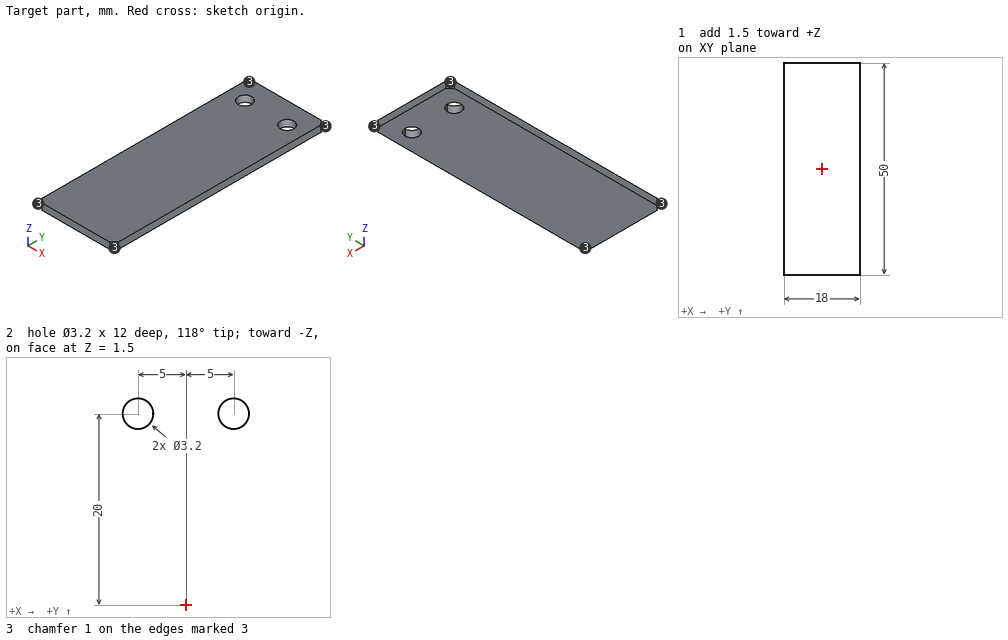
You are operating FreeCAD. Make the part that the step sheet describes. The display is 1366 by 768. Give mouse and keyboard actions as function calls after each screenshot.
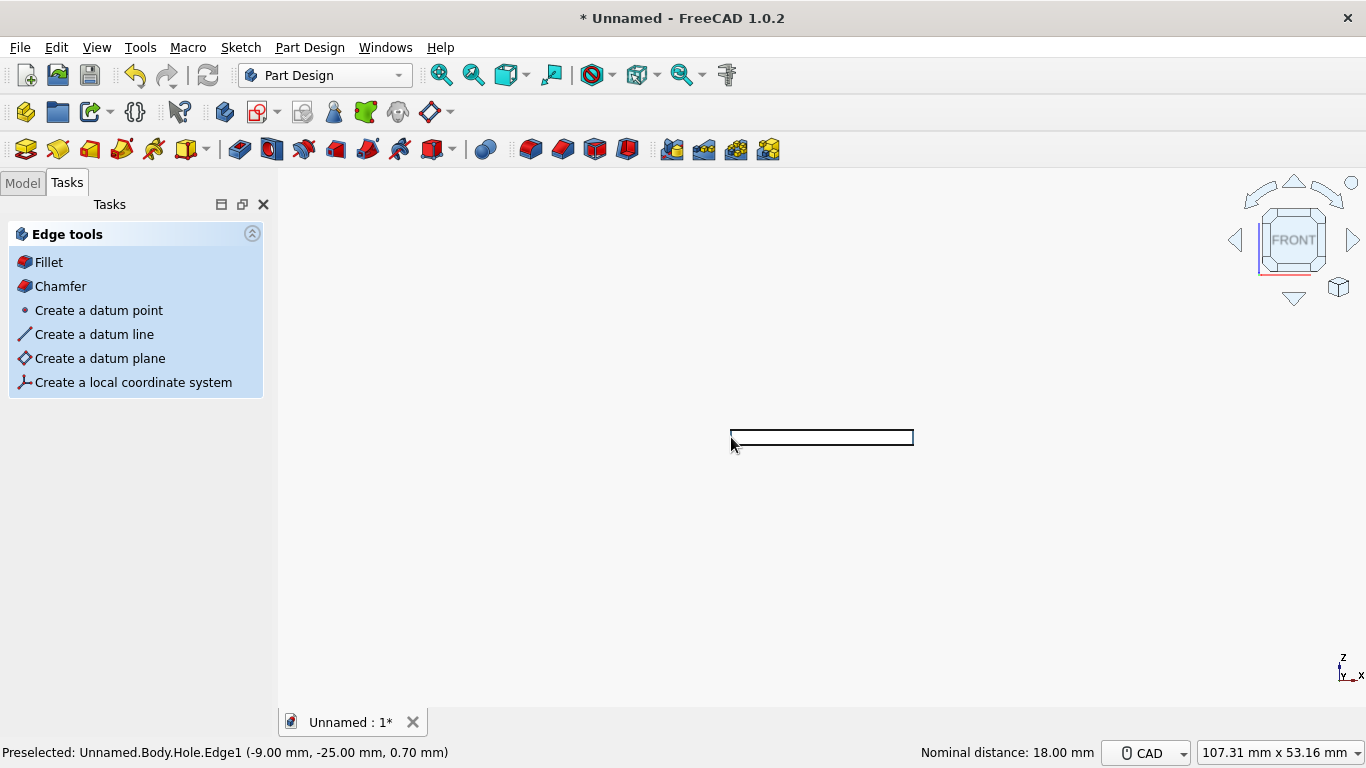
scroll(731, 437, up, 5)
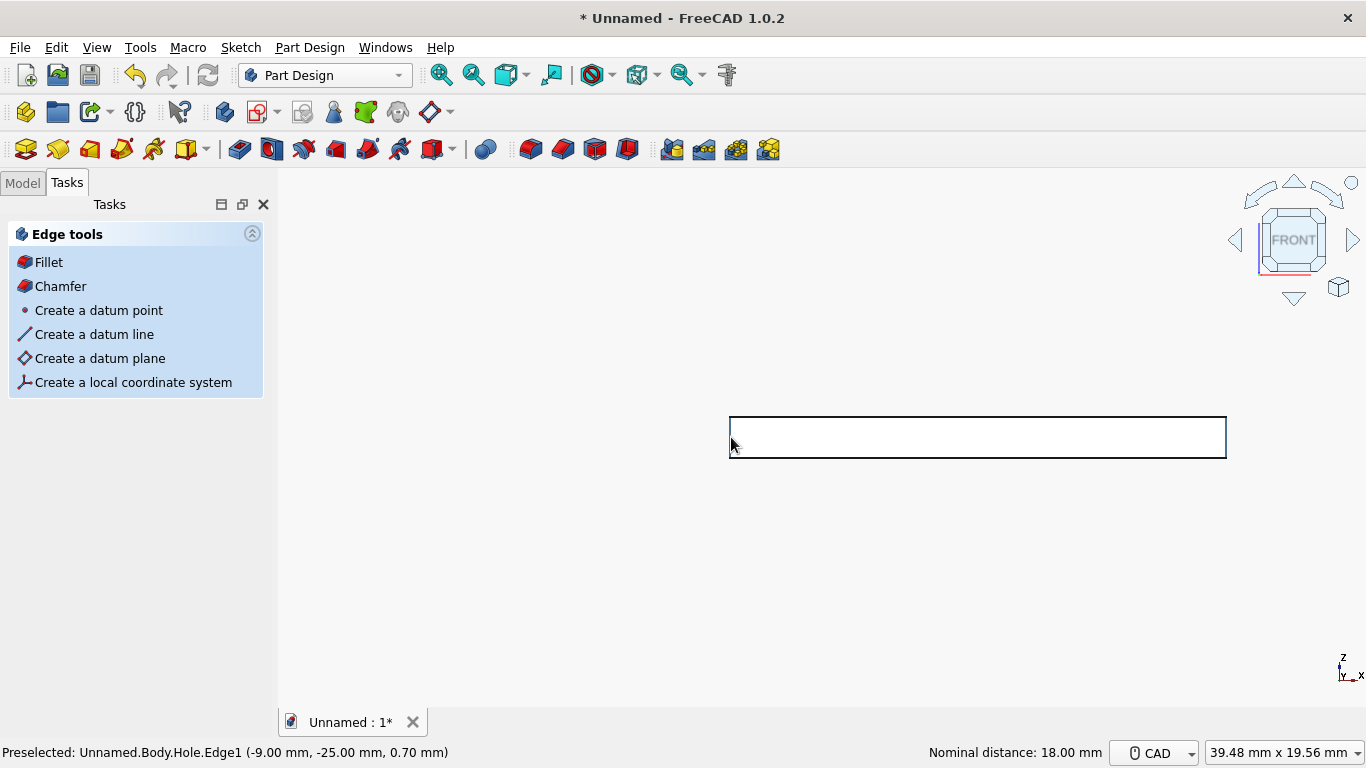
click(442, 76)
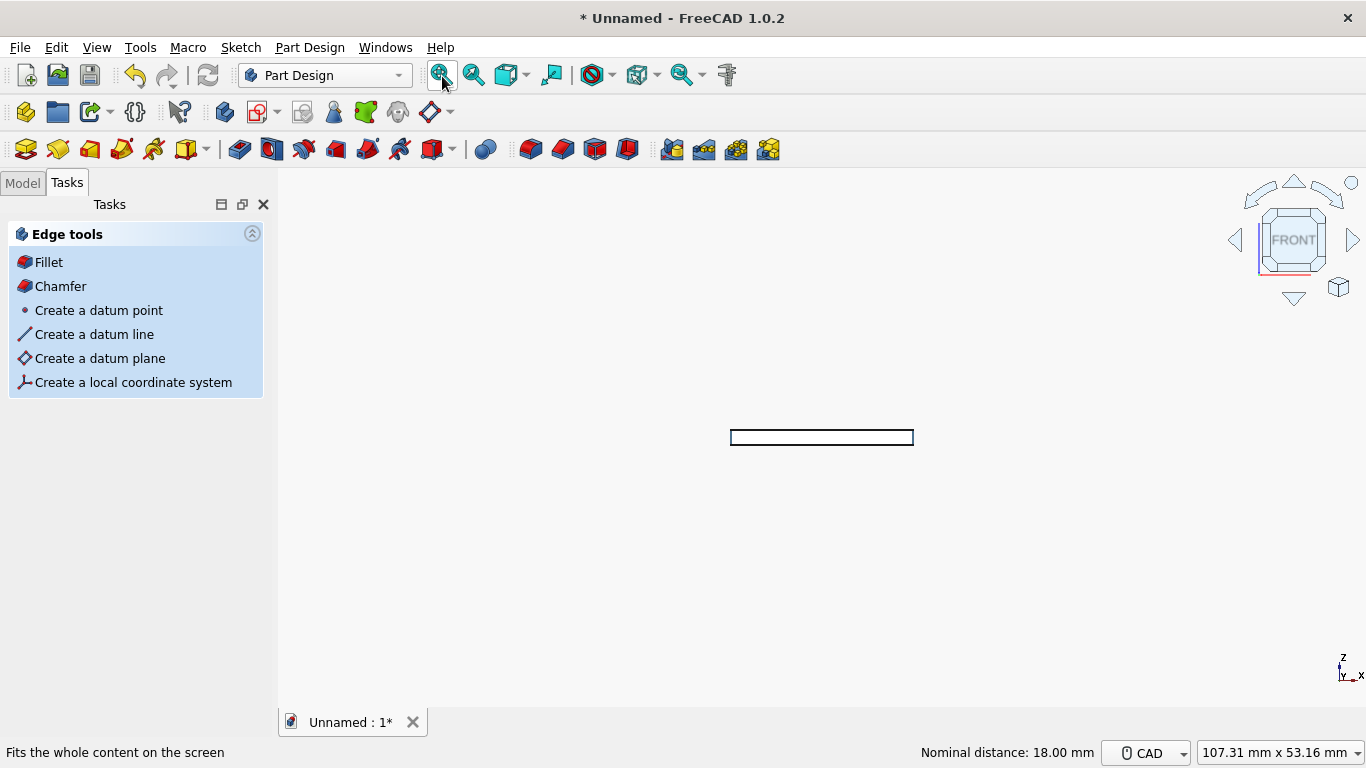
key(3)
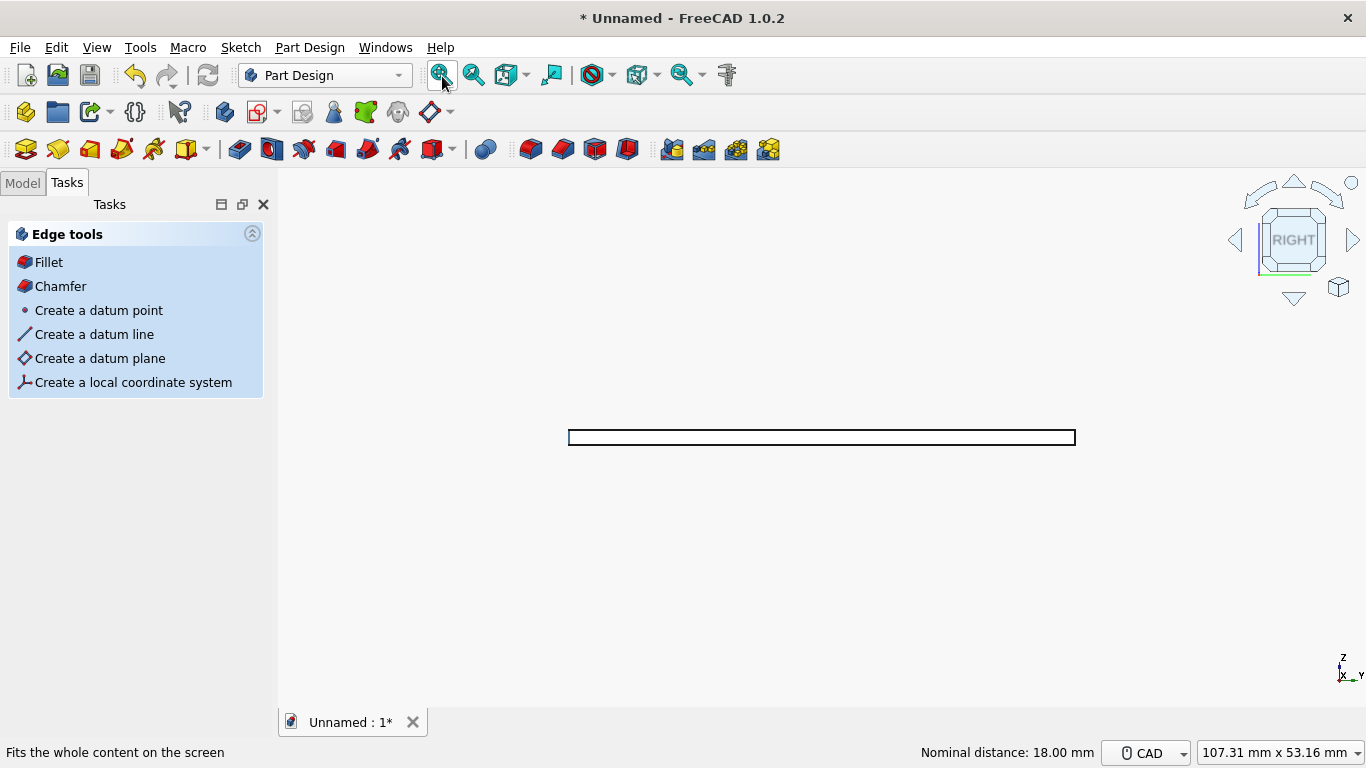
click(1075, 436, ctrl)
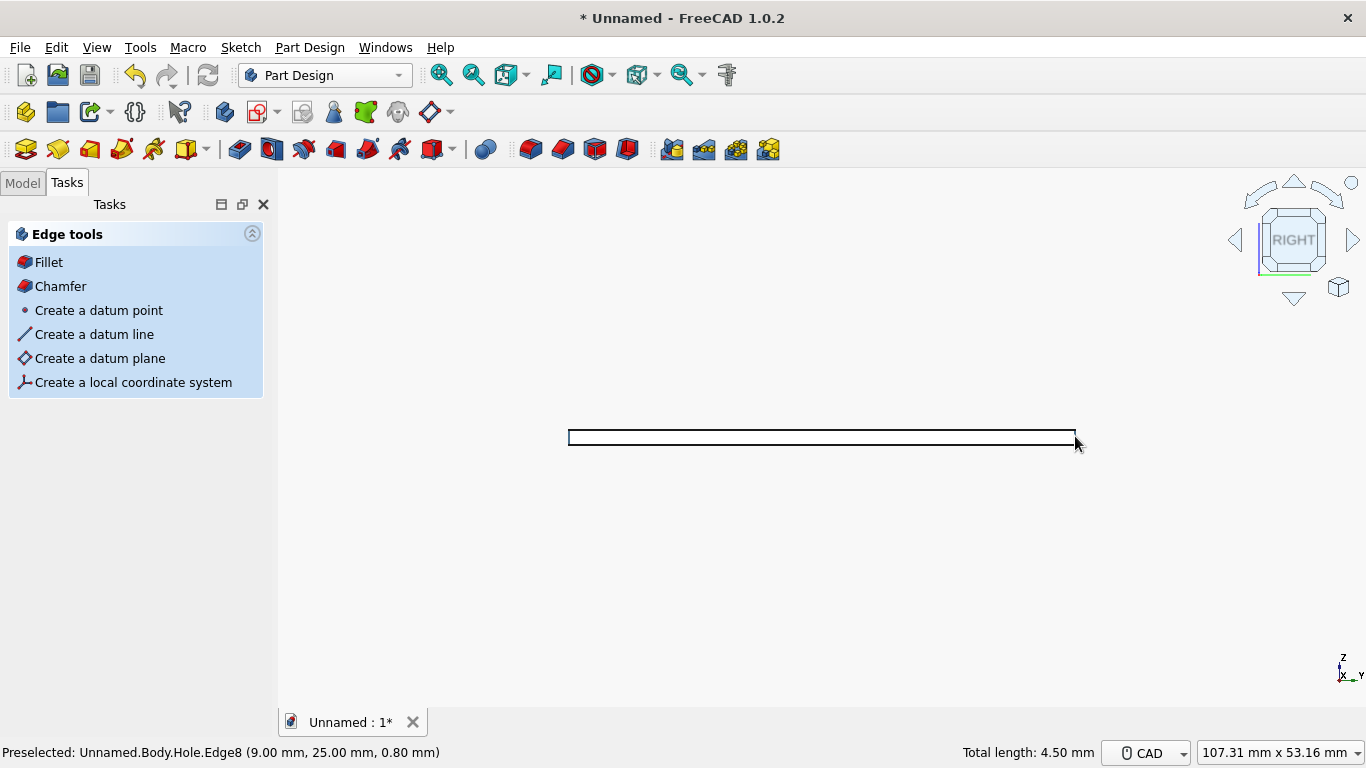
scroll(1075, 436, up, 5)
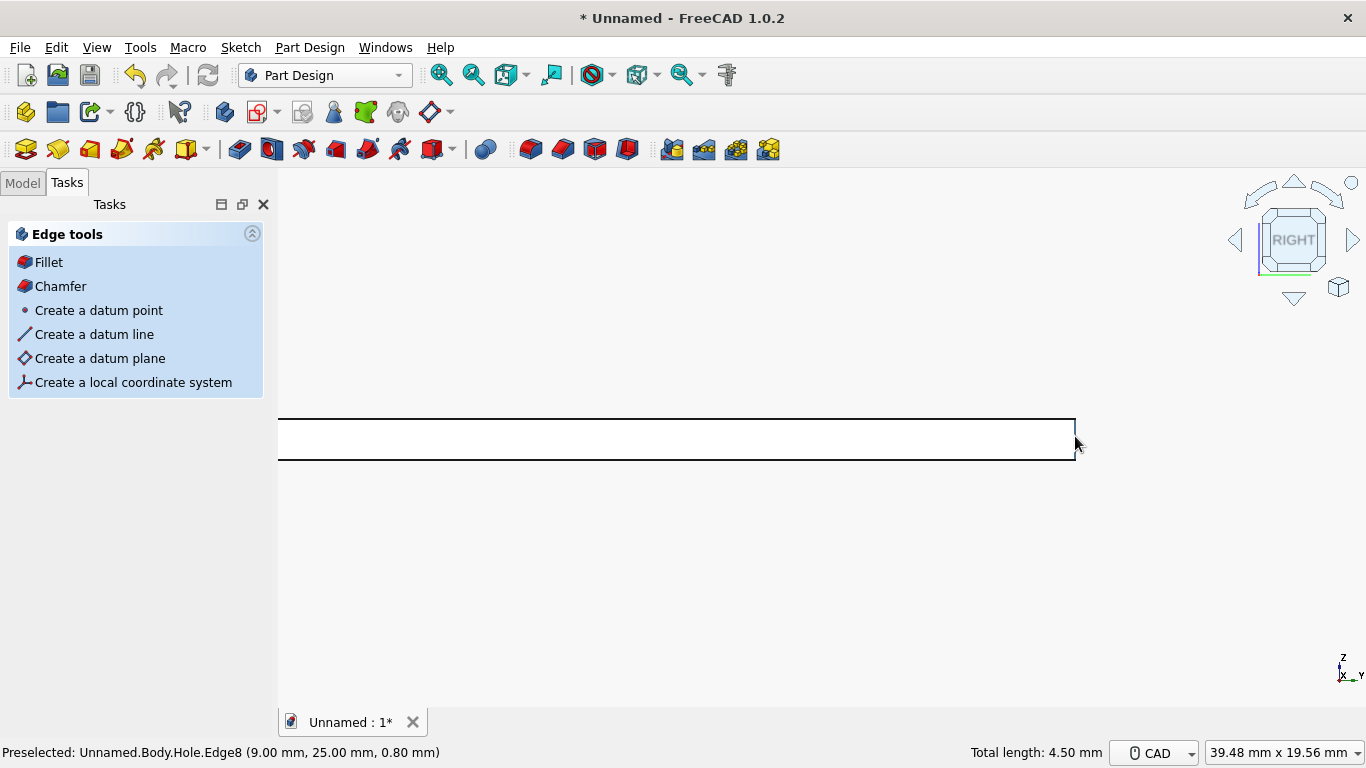
click(442, 76)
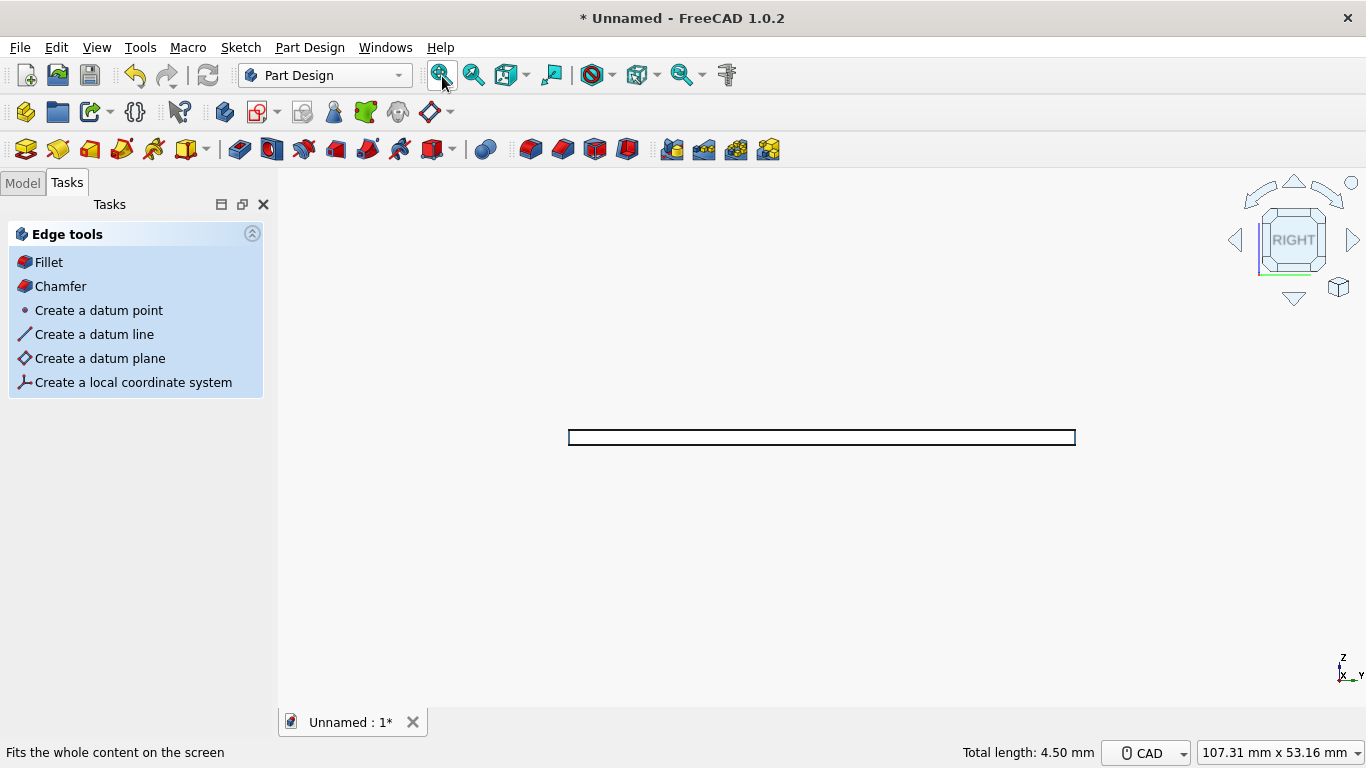
key(5)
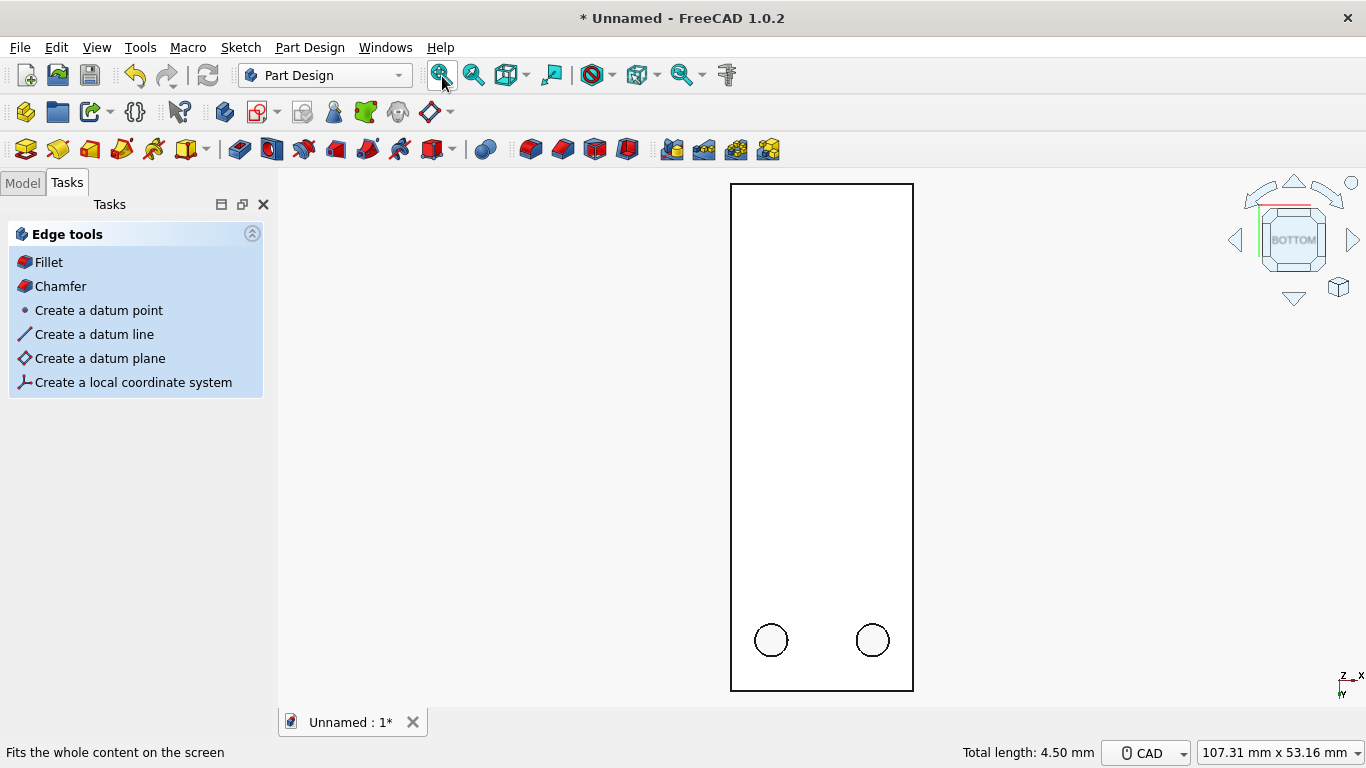
key(4)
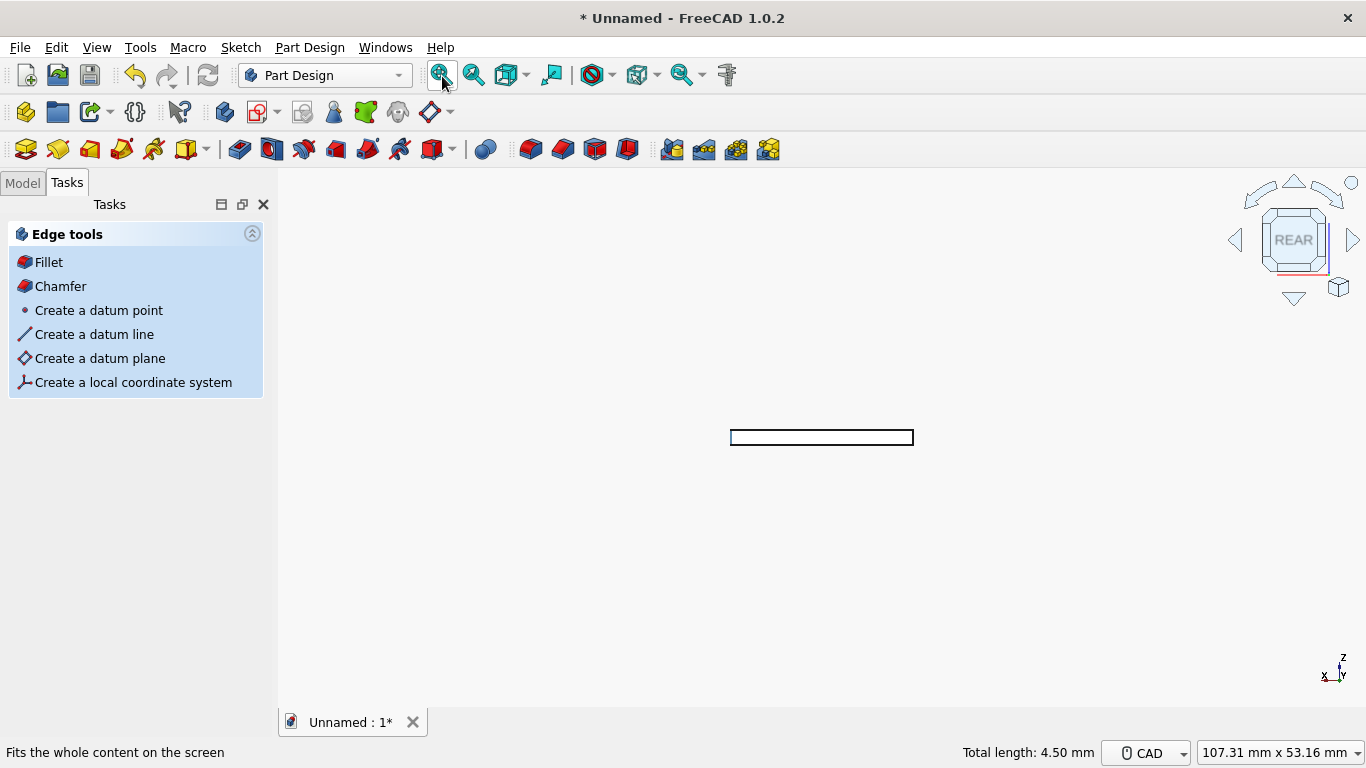
key(v)
key(f)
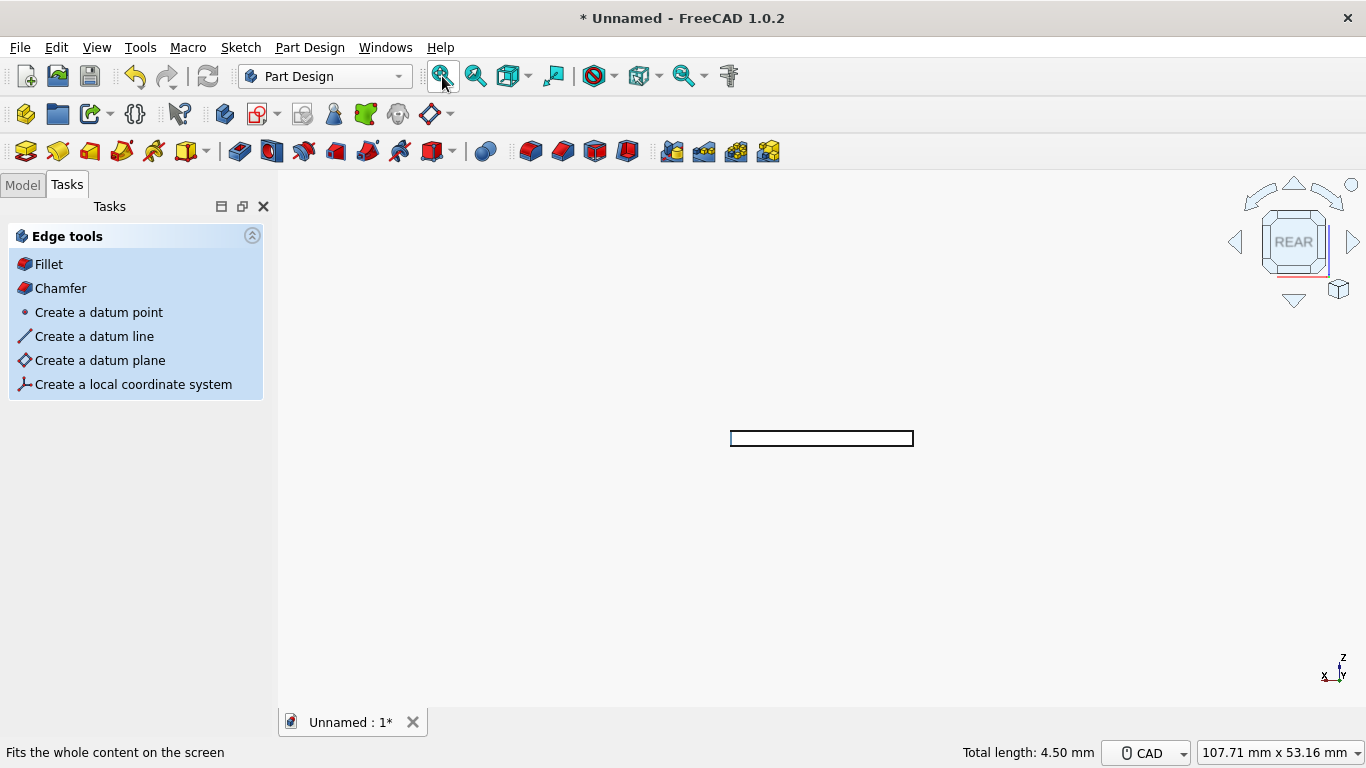
click(913, 438, ctrl)